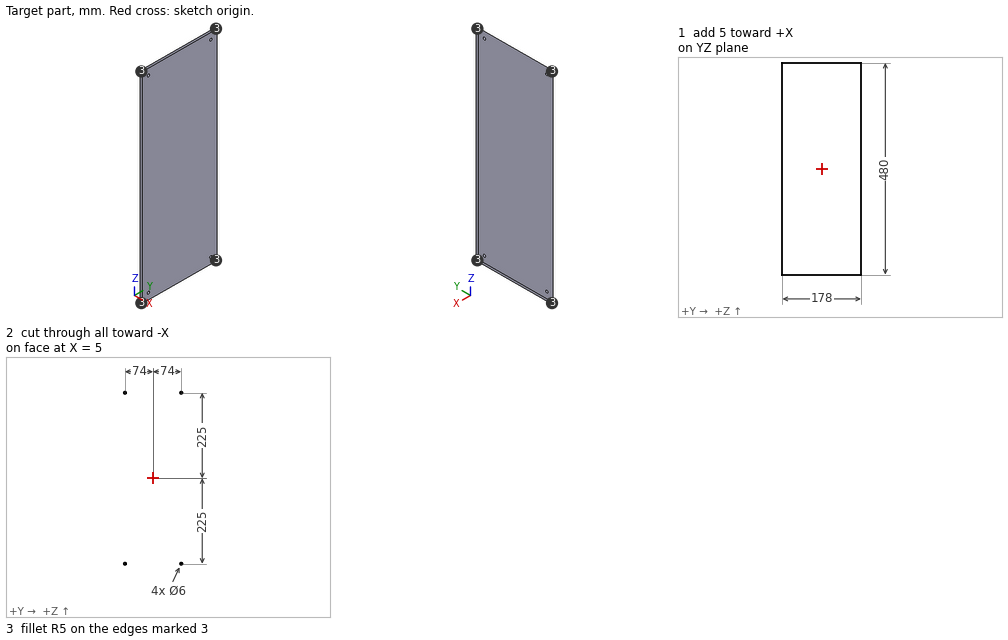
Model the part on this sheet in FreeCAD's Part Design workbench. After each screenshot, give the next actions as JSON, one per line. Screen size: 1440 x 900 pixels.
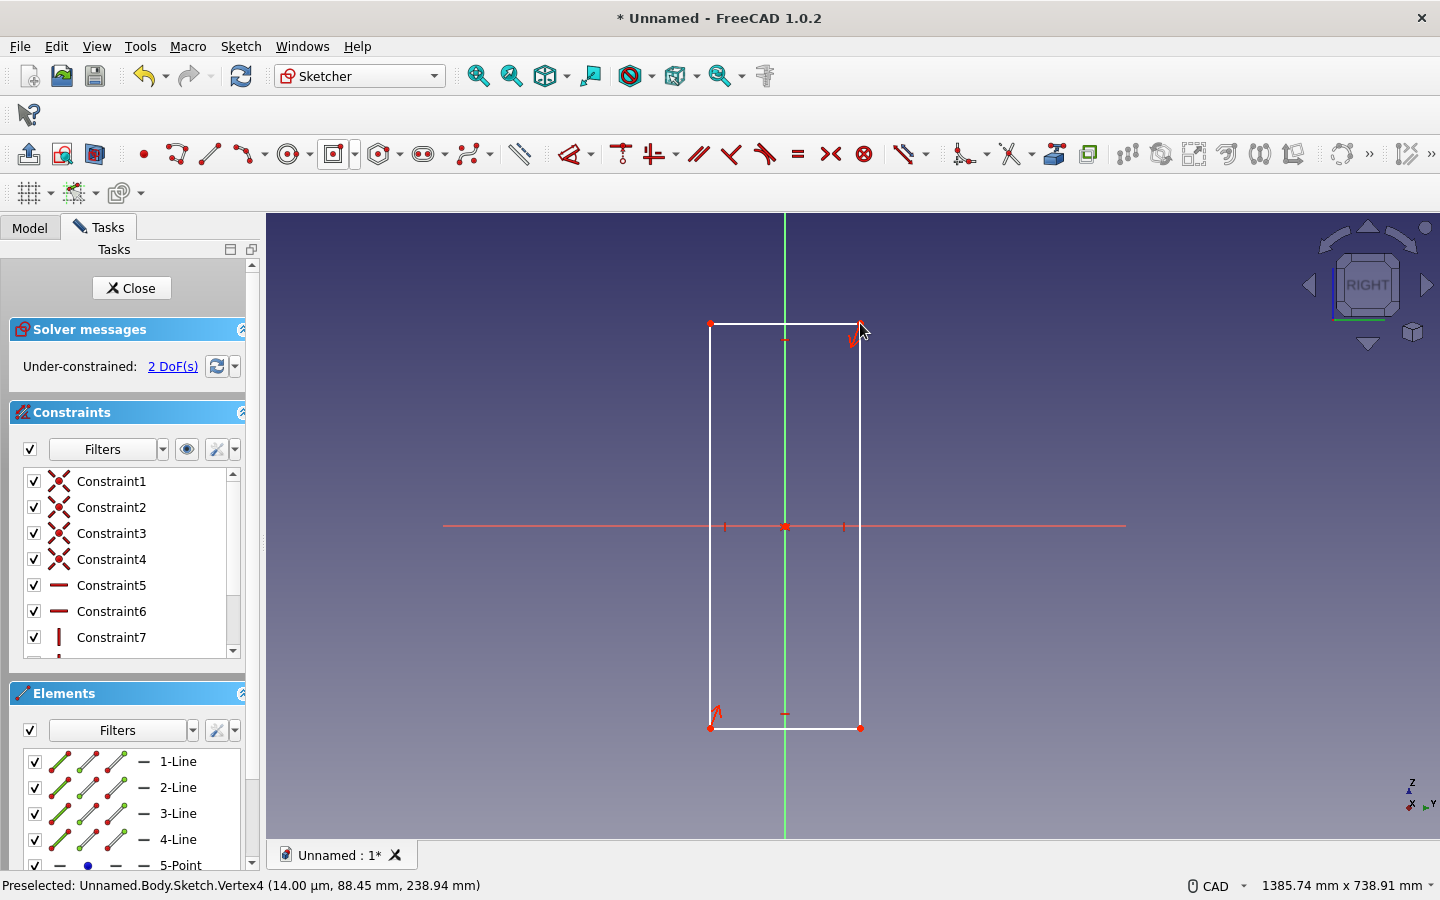
{"action": "left_click", "coordinate": [755, 729]}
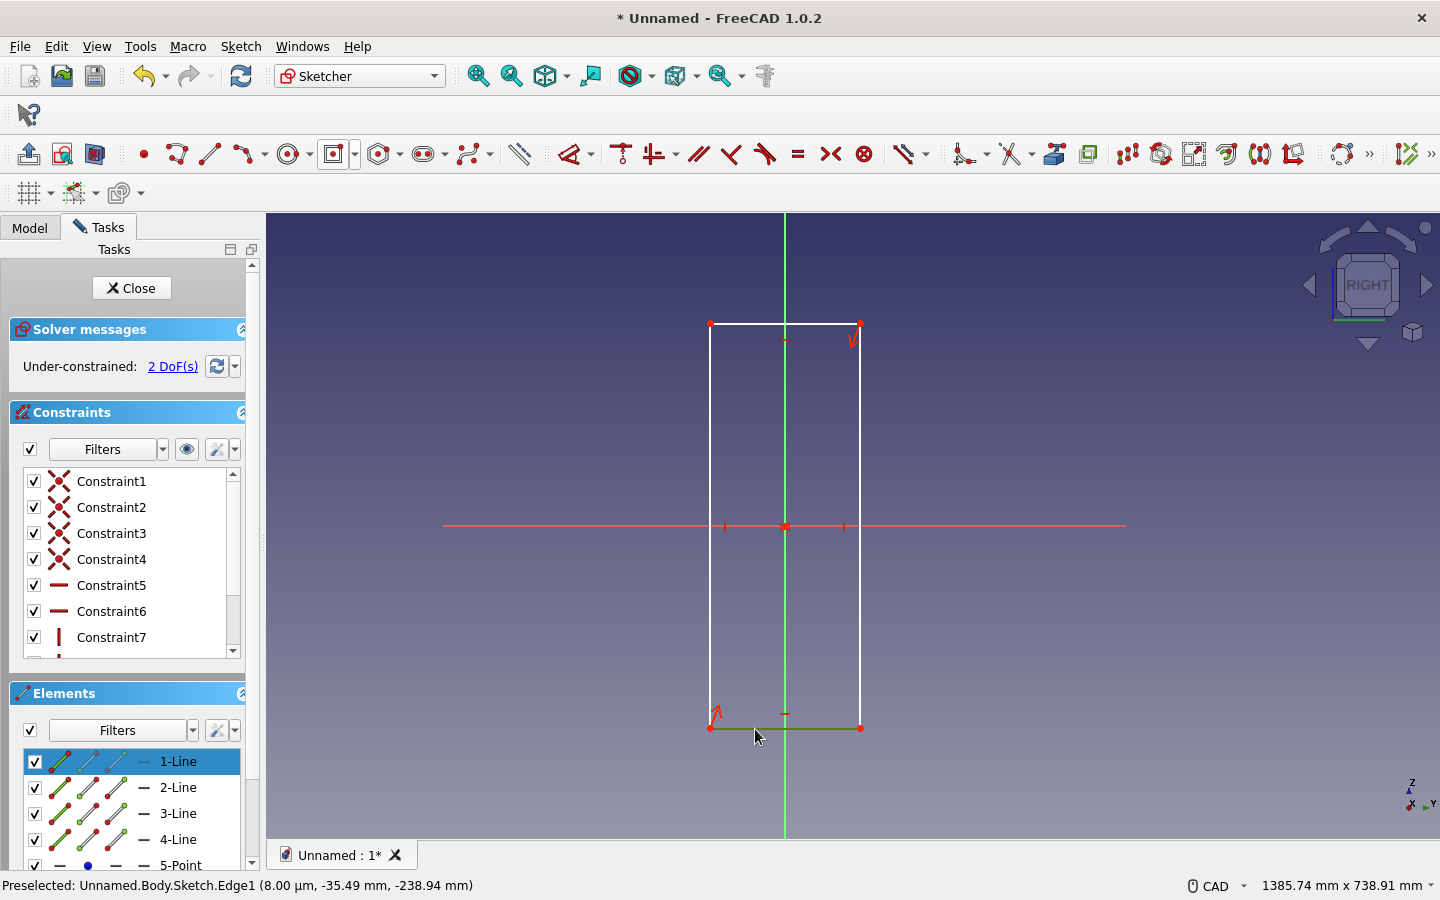
{"action": "key", "text": "l"}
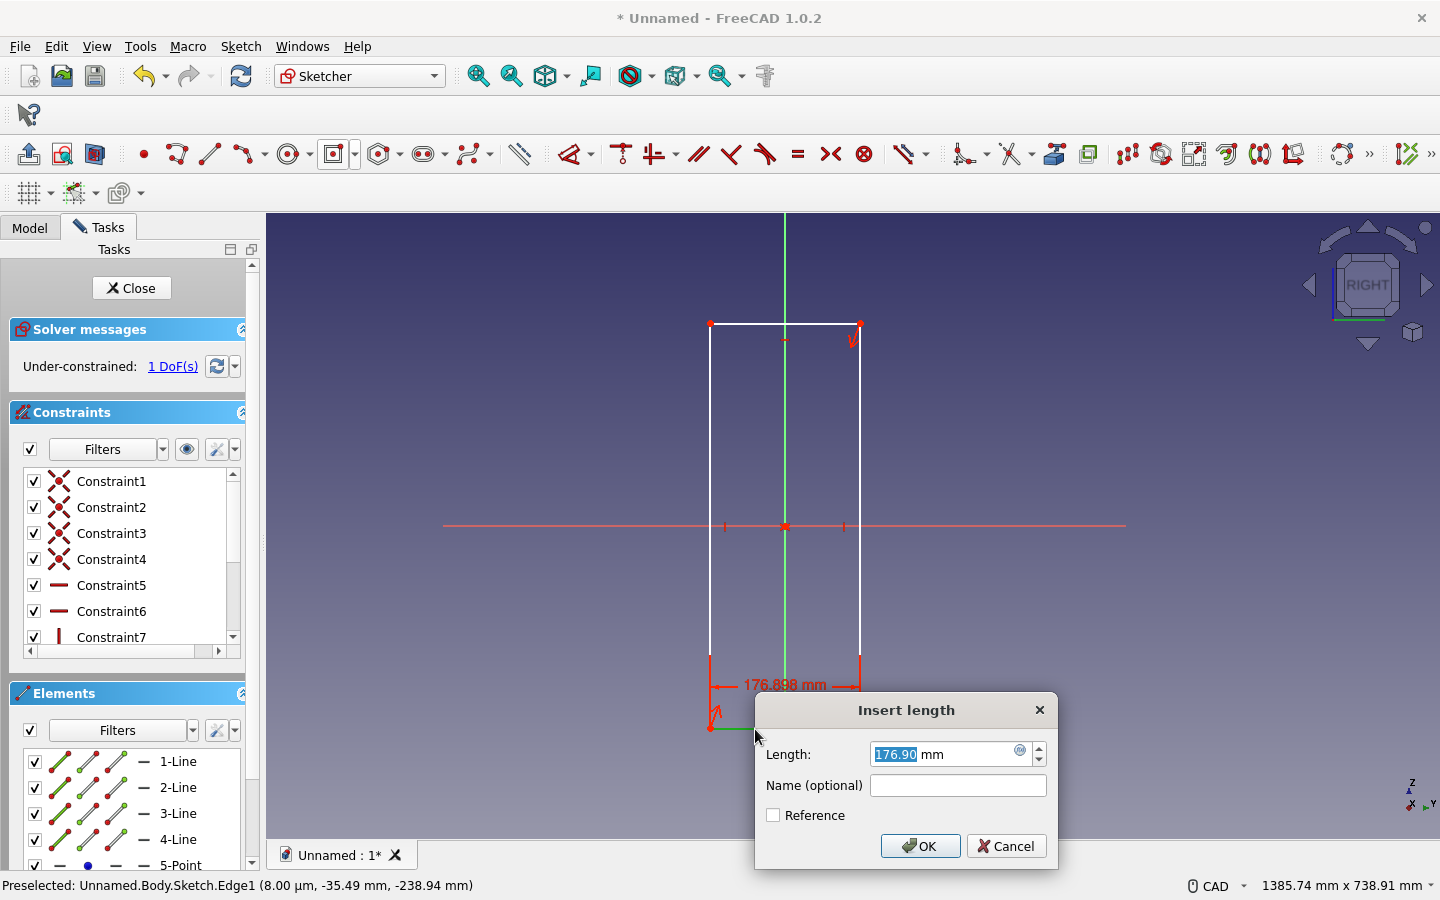
{"action": "type", "text": "178"}
{"action": "key", "text": "Return"}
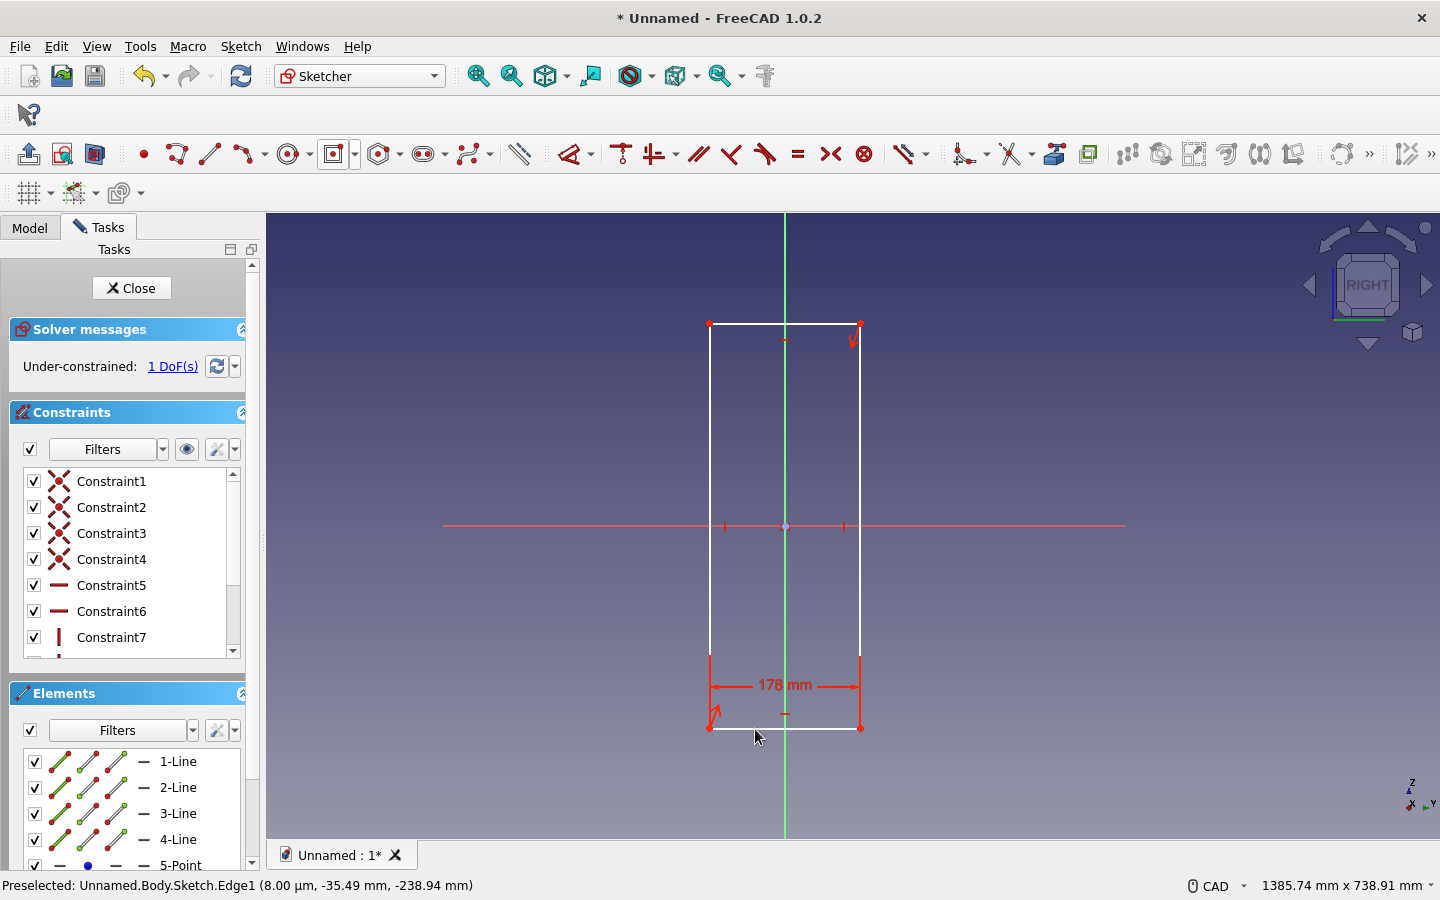
{"action": "left_click", "coordinate": [860, 607]}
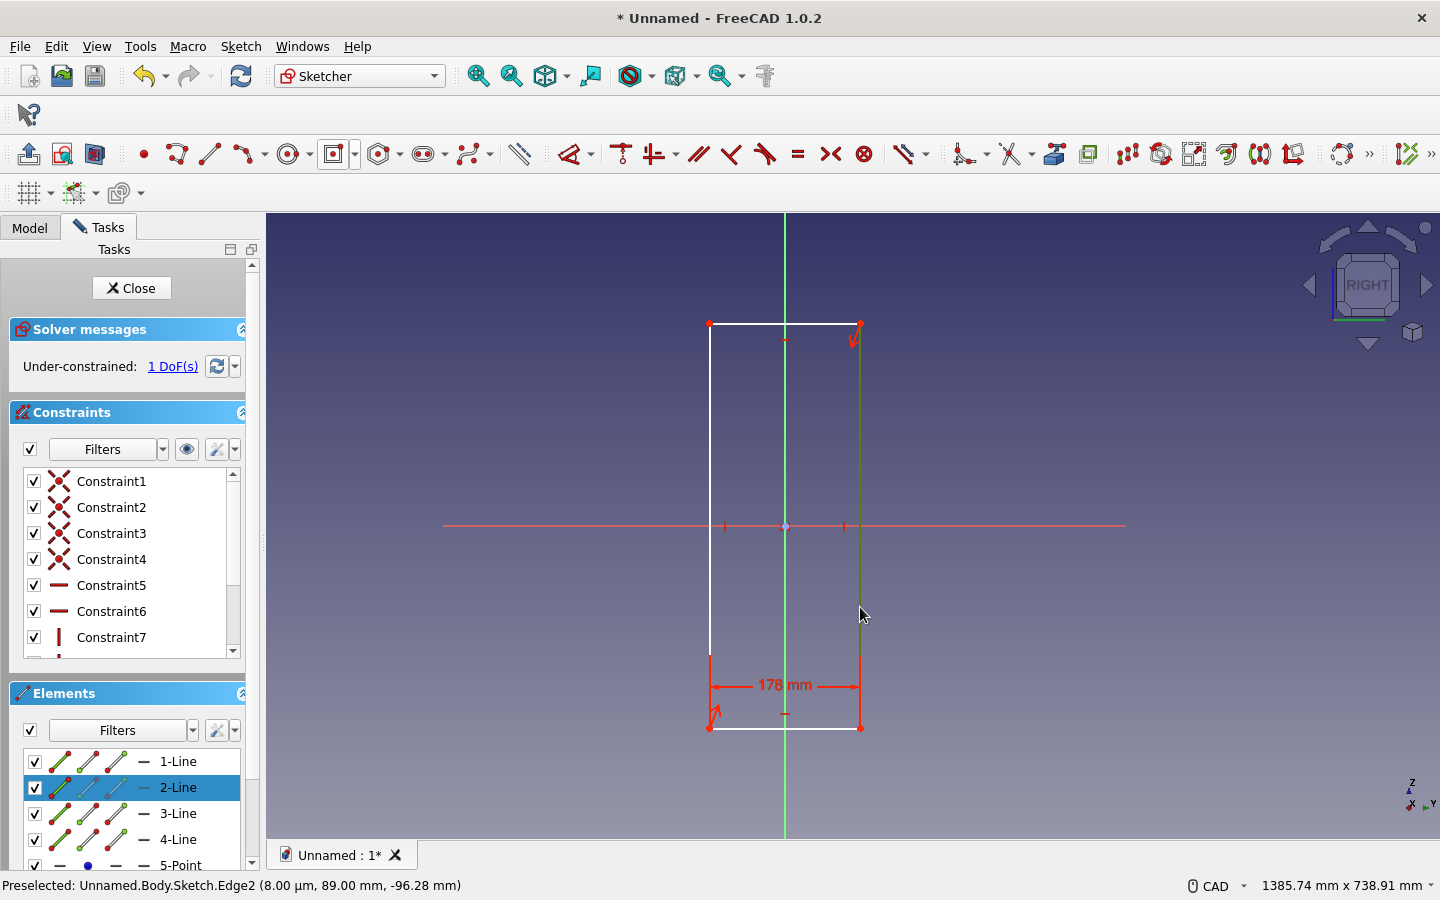
{"action": "key", "text": "i"}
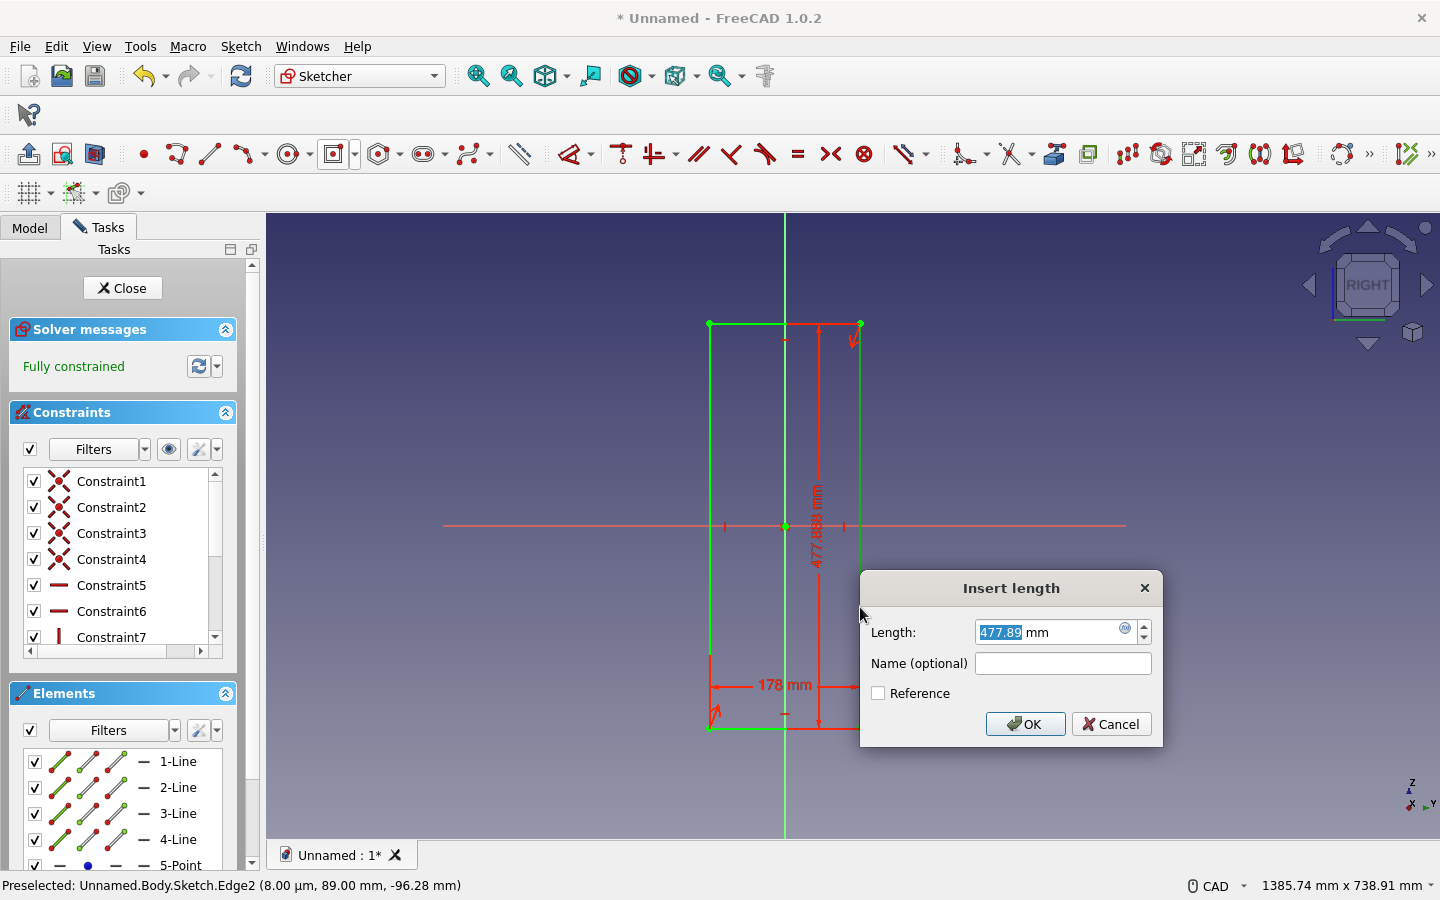
{"action": "type", "text": "480"}
{"action": "key", "text": "Return"}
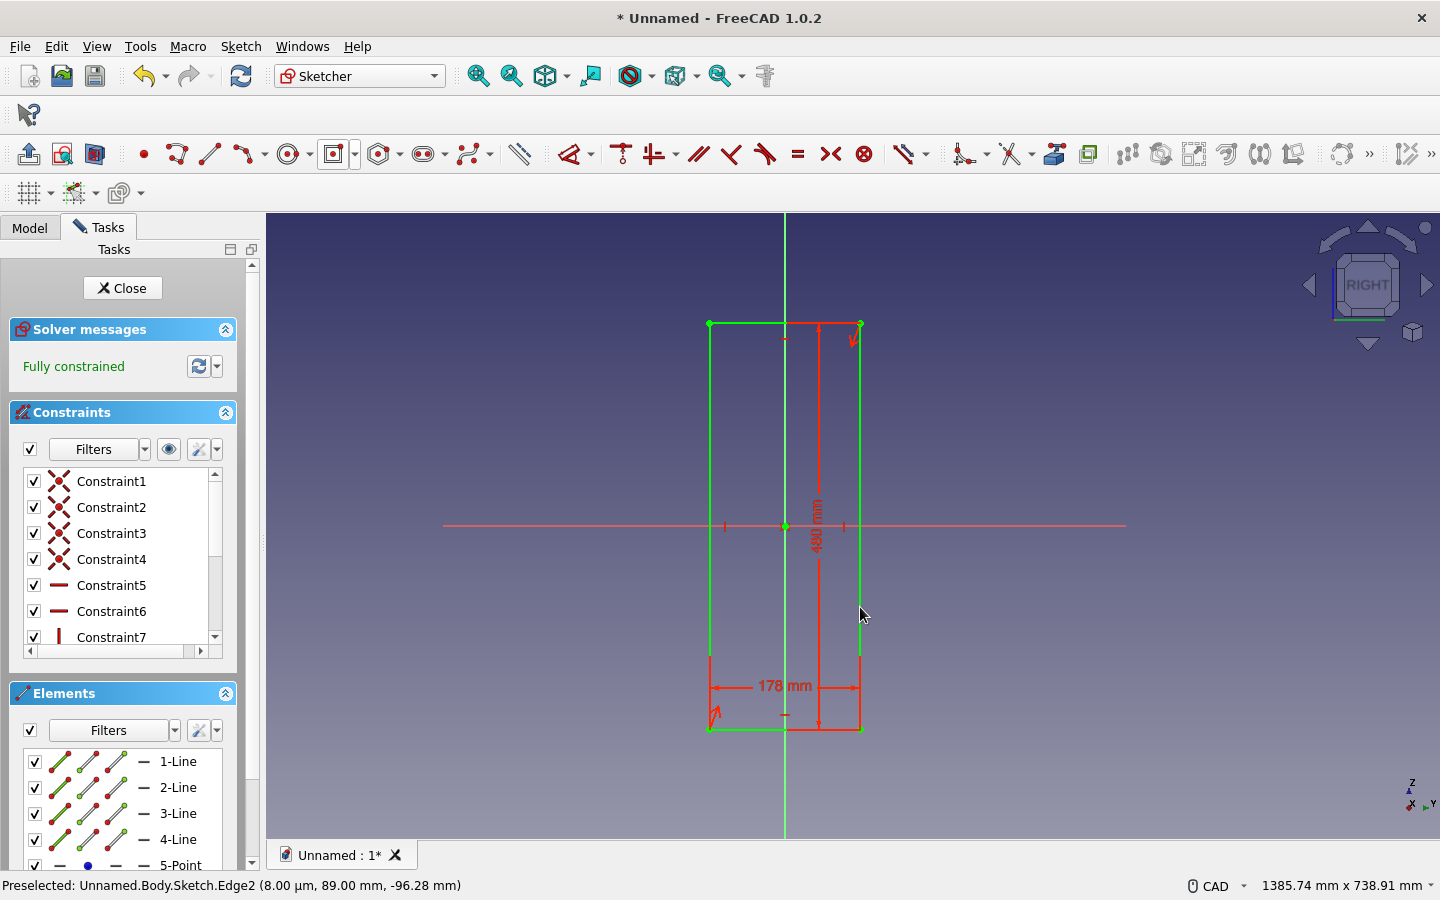
{"action": "left_click", "coordinate": [123, 288]}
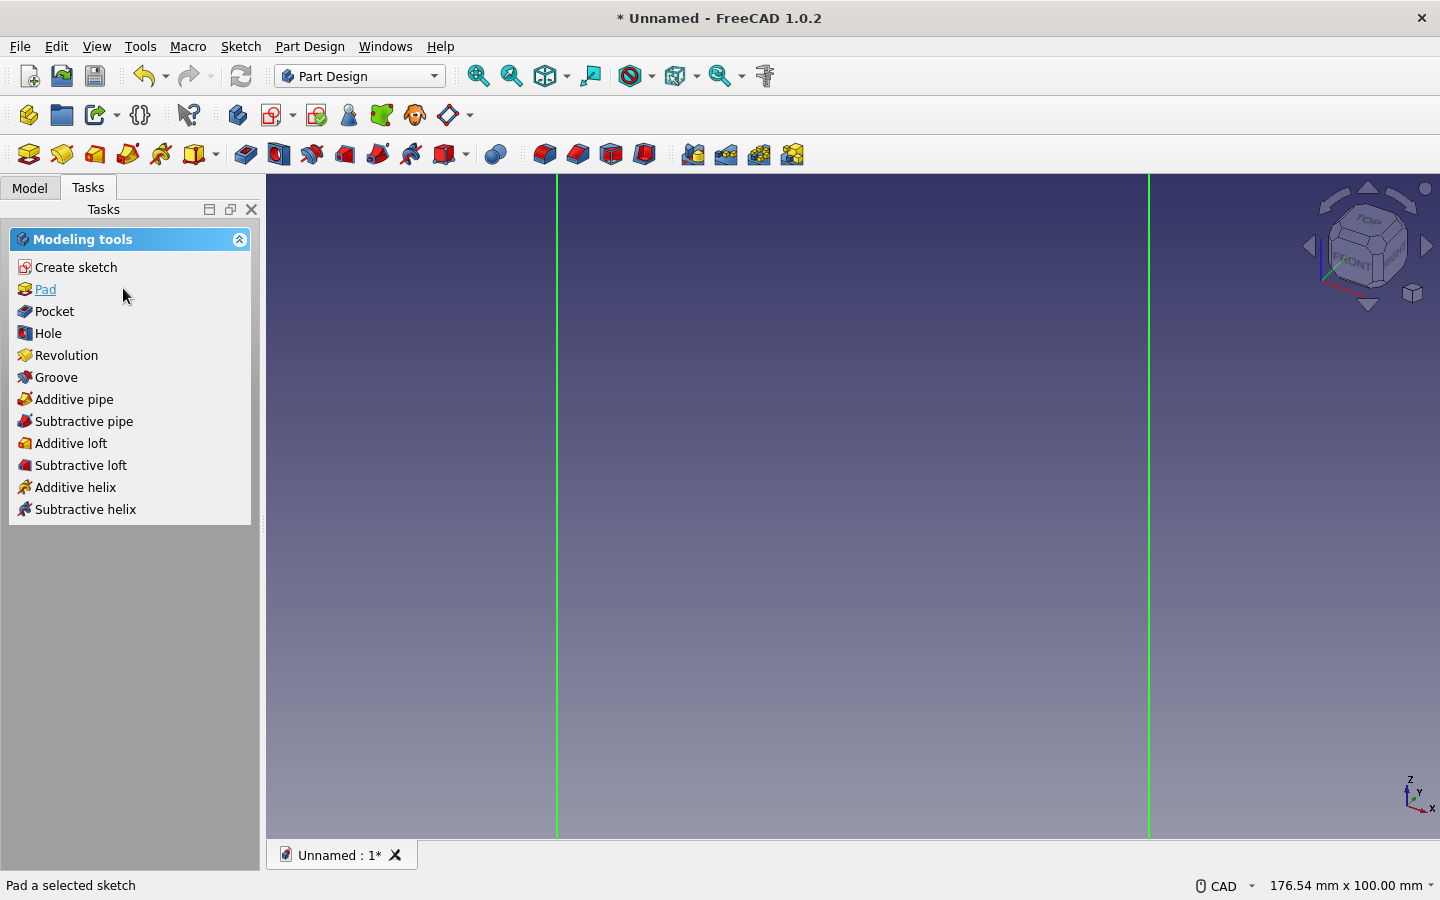
{"action": "left_click", "coordinate": [29, 154]}